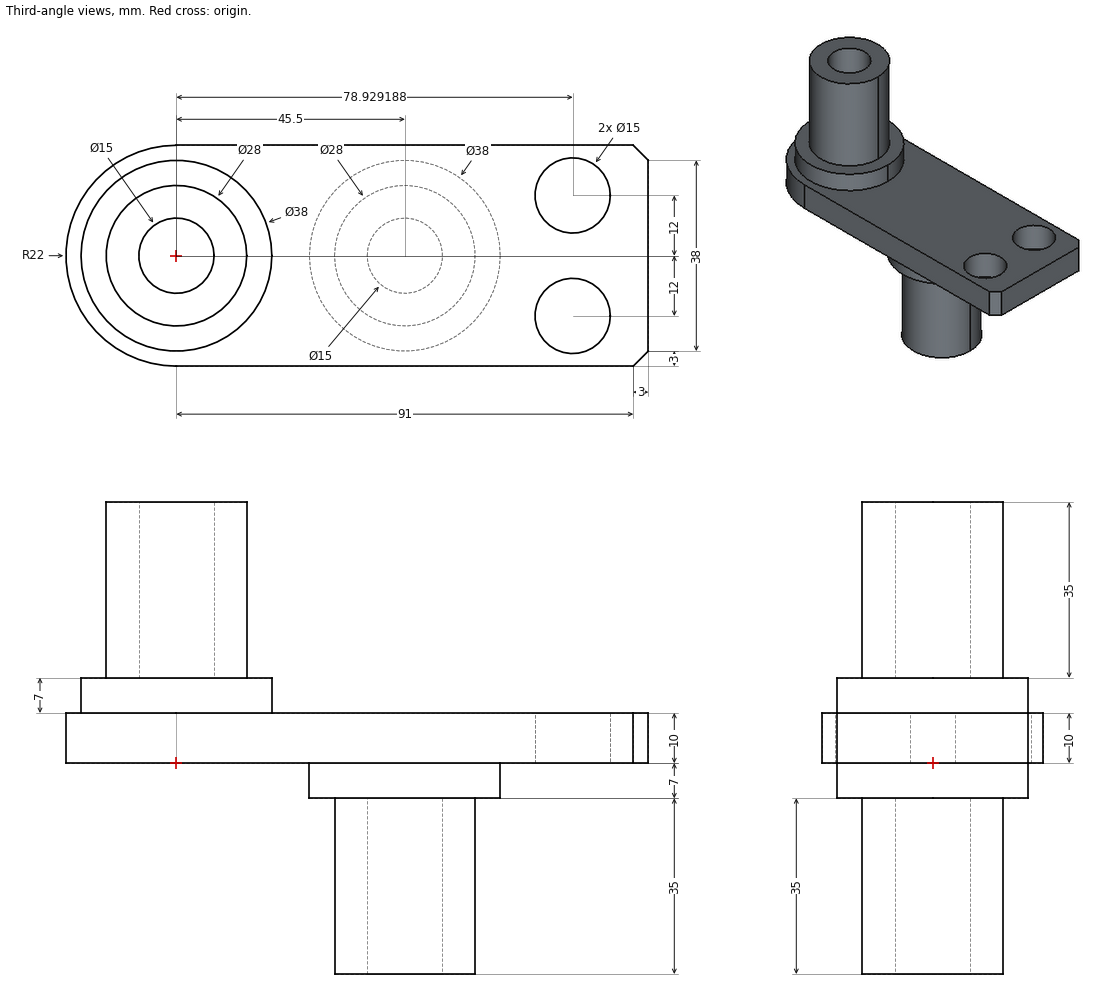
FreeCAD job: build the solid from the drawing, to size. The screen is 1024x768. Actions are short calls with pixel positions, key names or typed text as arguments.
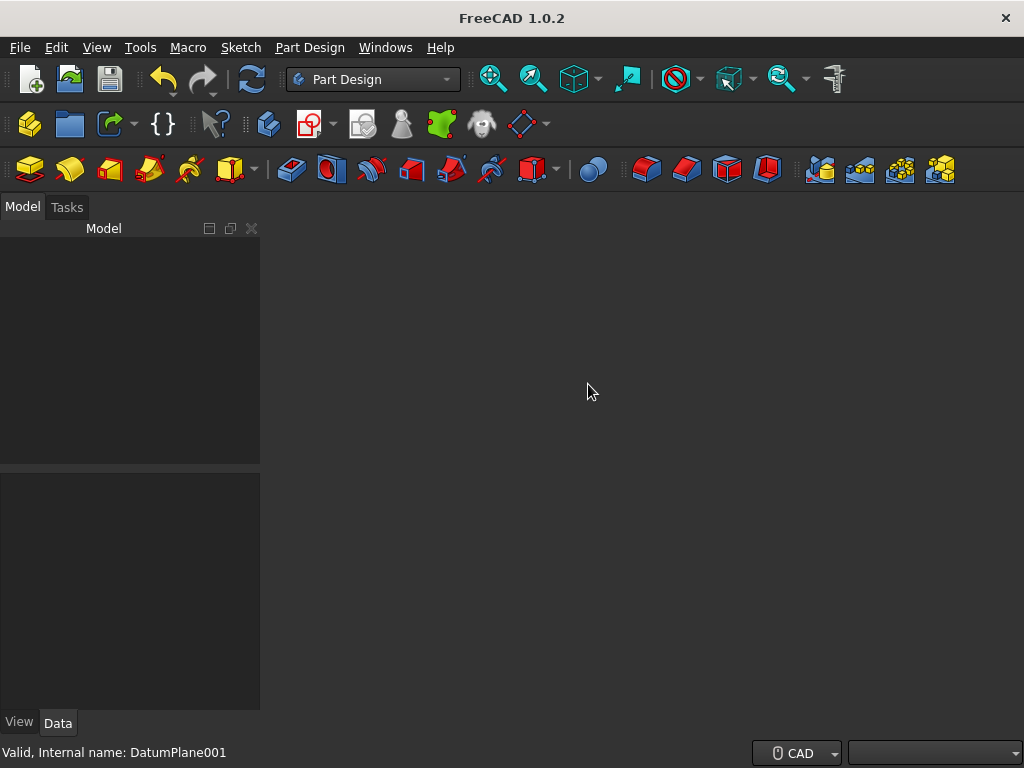
click(30, 80)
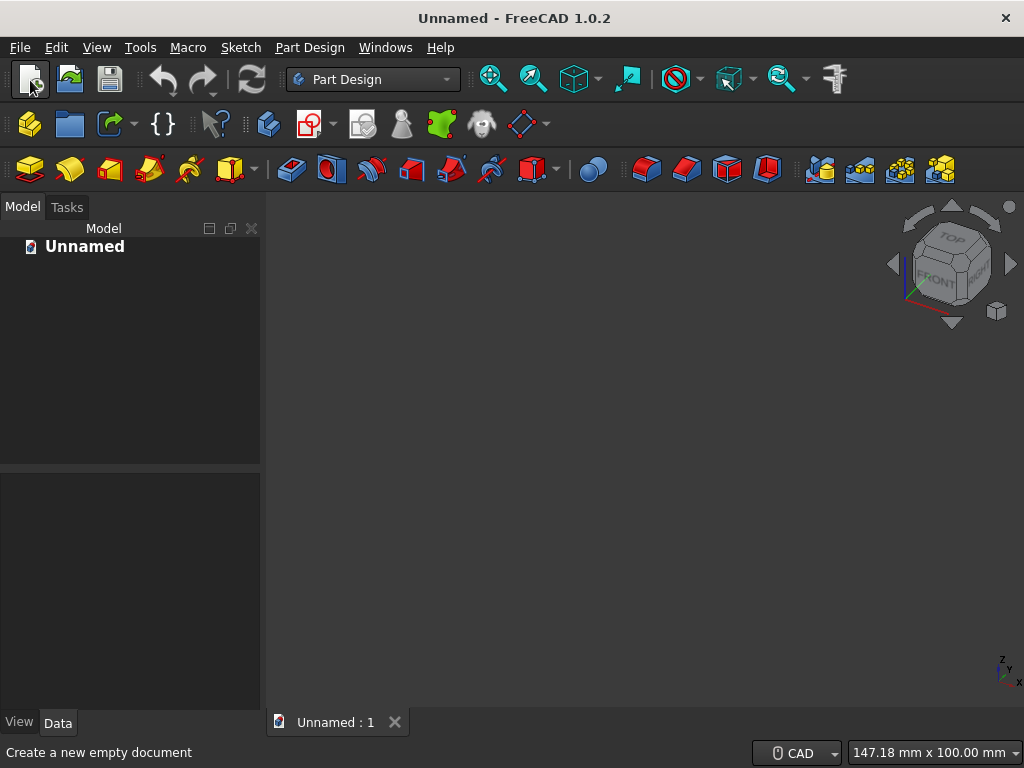
click(310, 124)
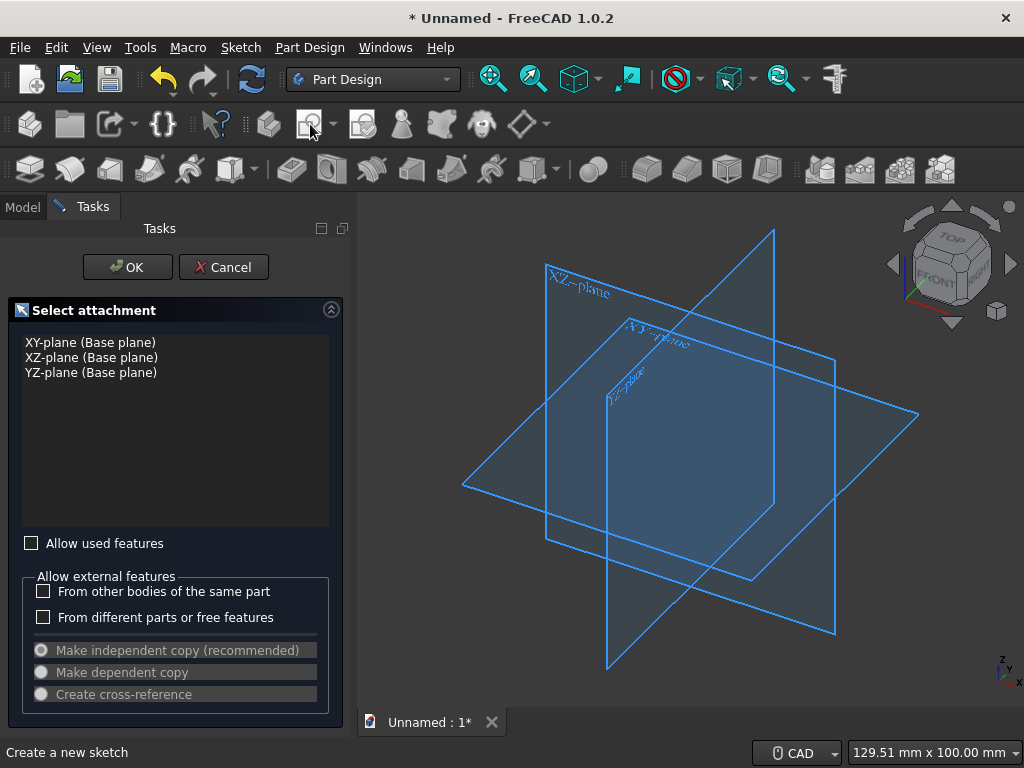
click(82, 342)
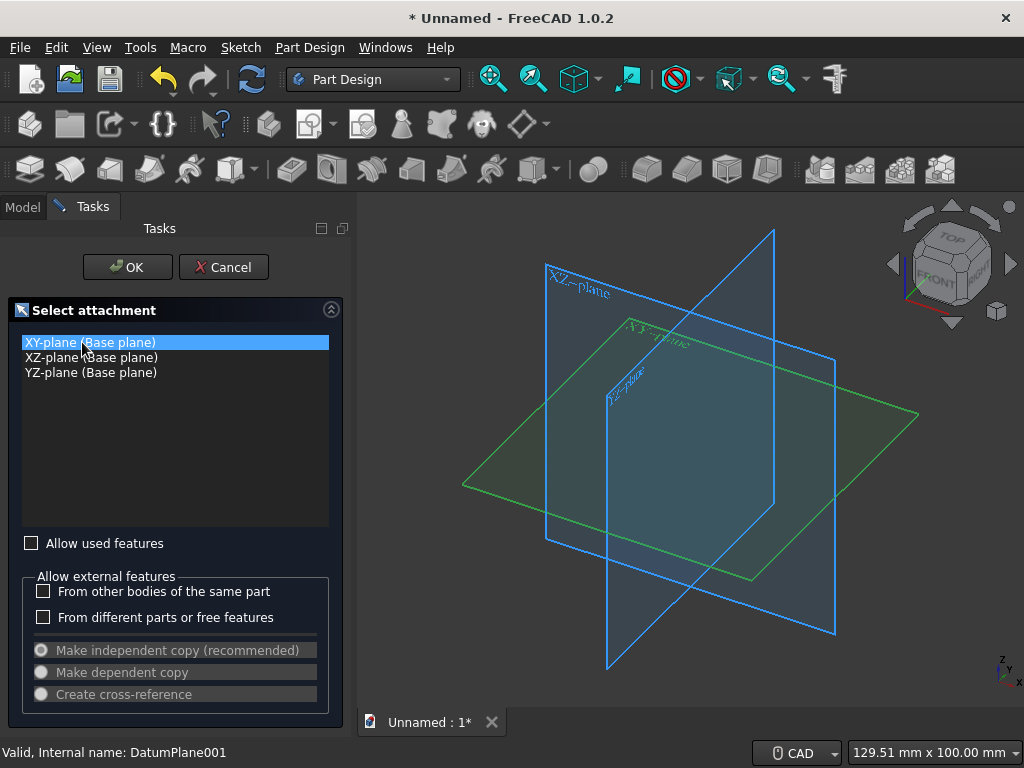
click(128, 267)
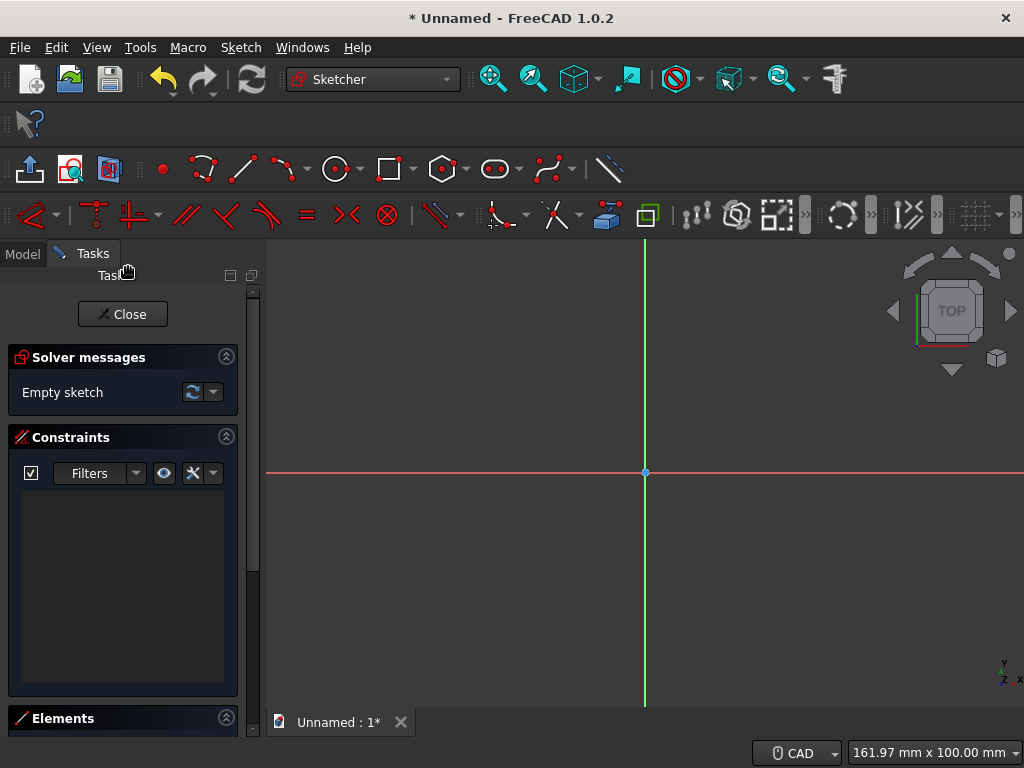
scroll(294, 473, down, 2)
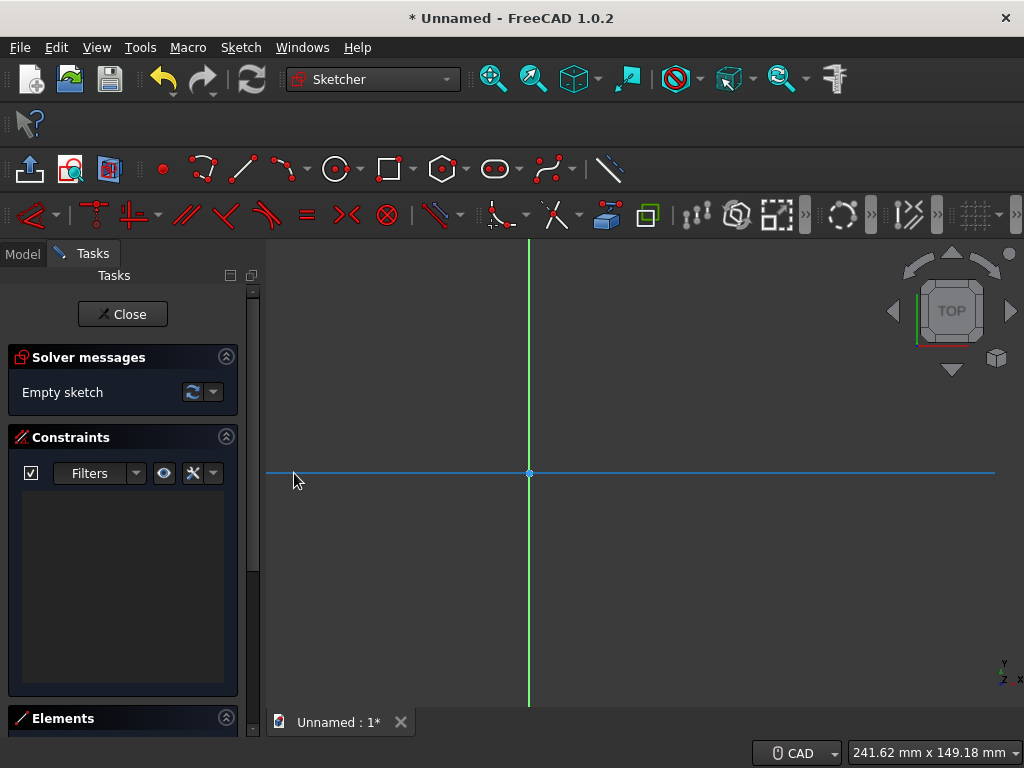
click(204, 170)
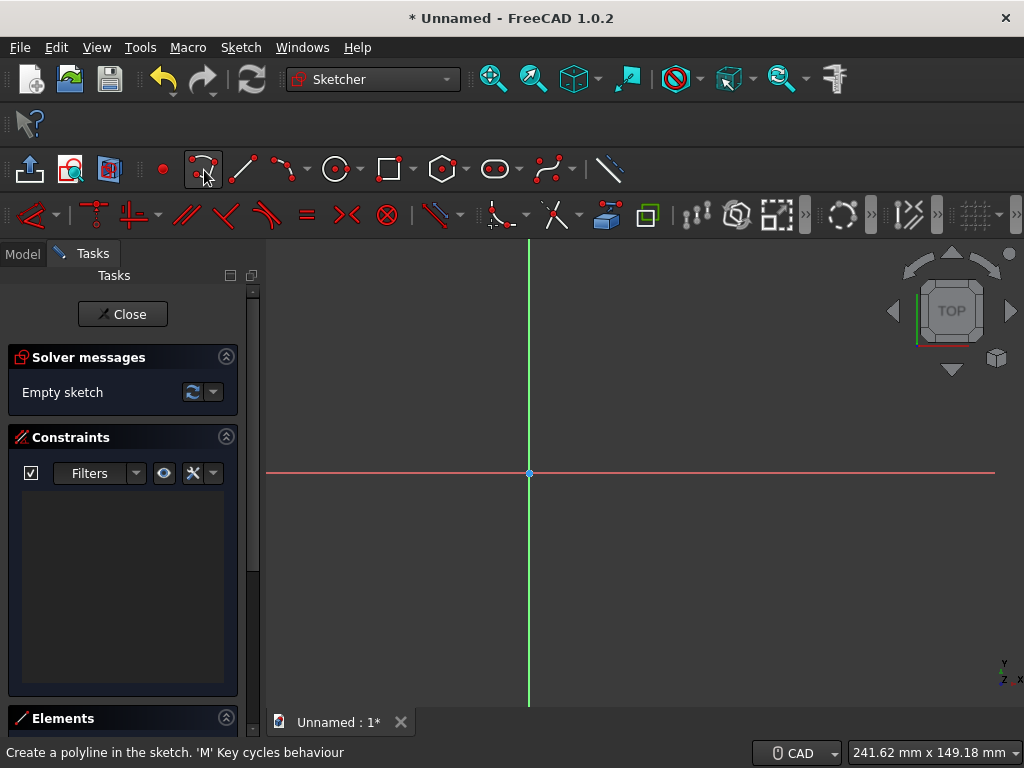
click(529, 542)
click(815, 542)
click(824, 533)
click(824, 414)
click(815, 404)
click(529, 404)
right_click(529, 404)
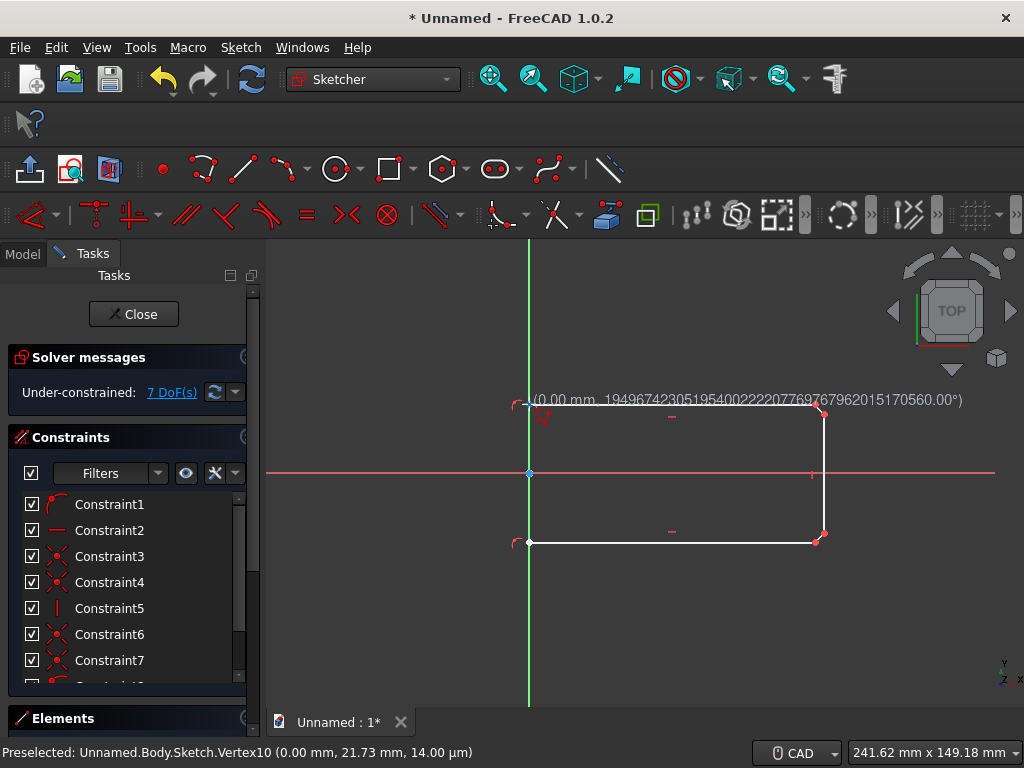
click(284, 170)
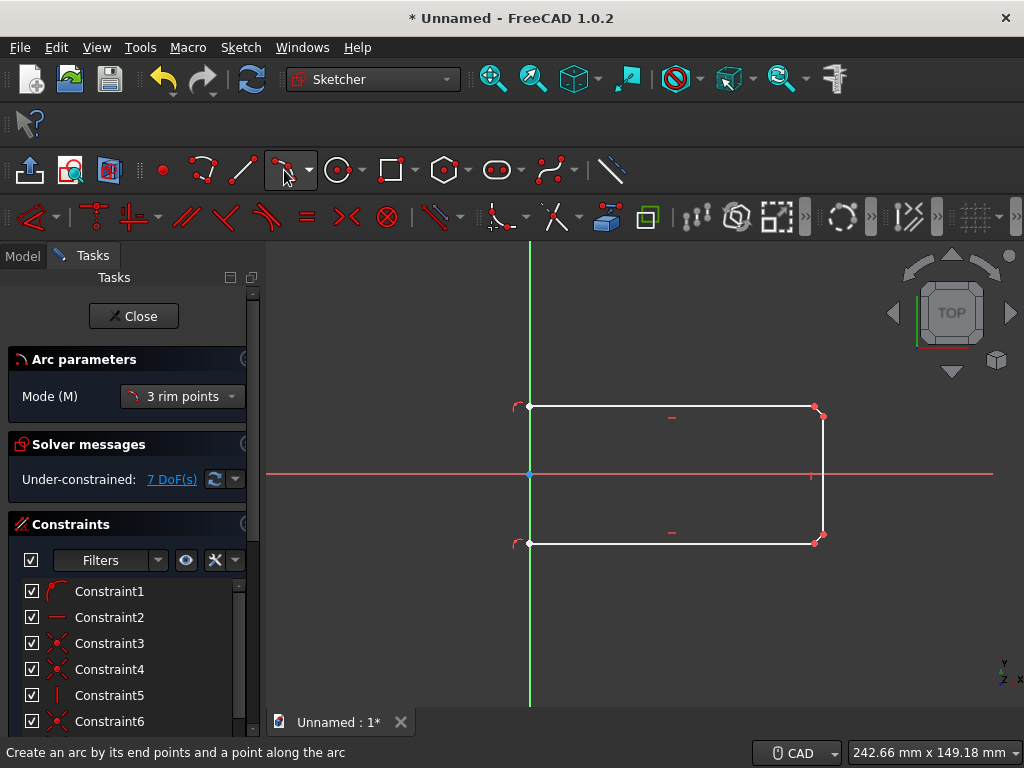
click(530, 406)
click(530, 544)
click(464, 453)
key(Escape)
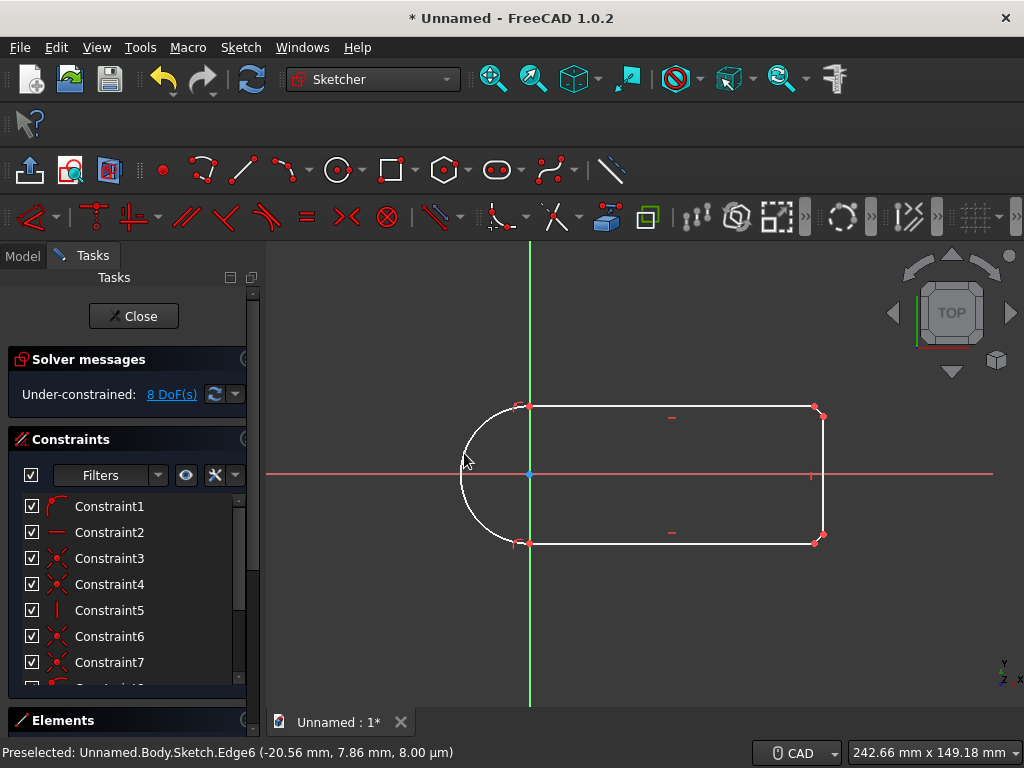
click(615, 544)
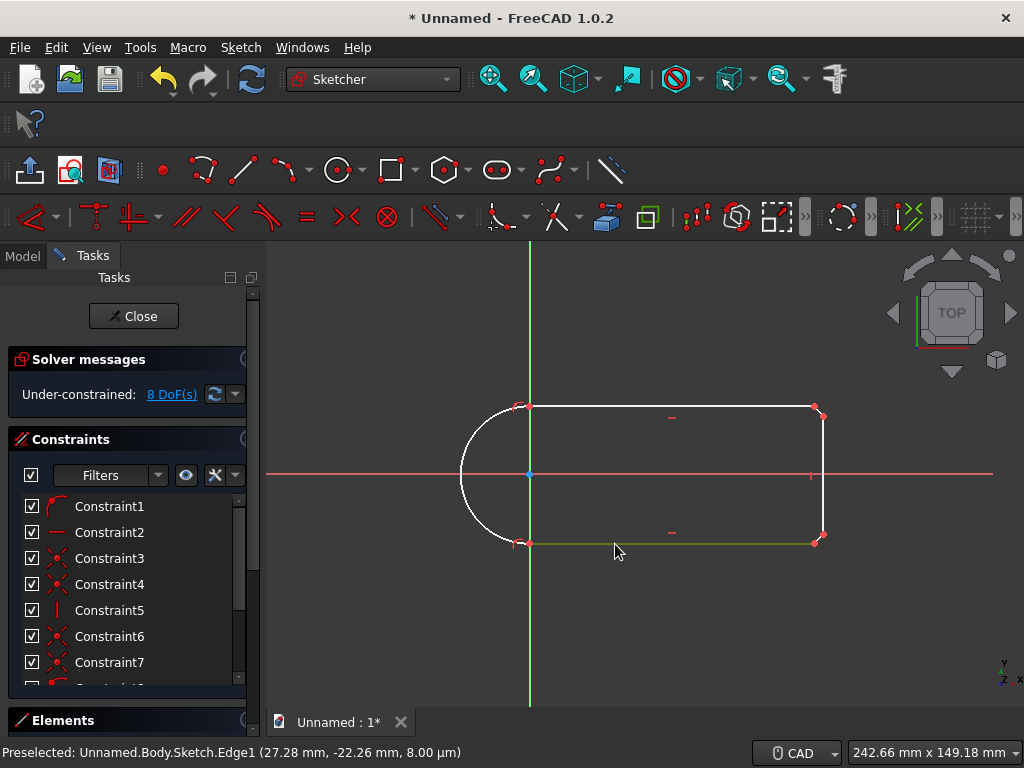
click(474, 434)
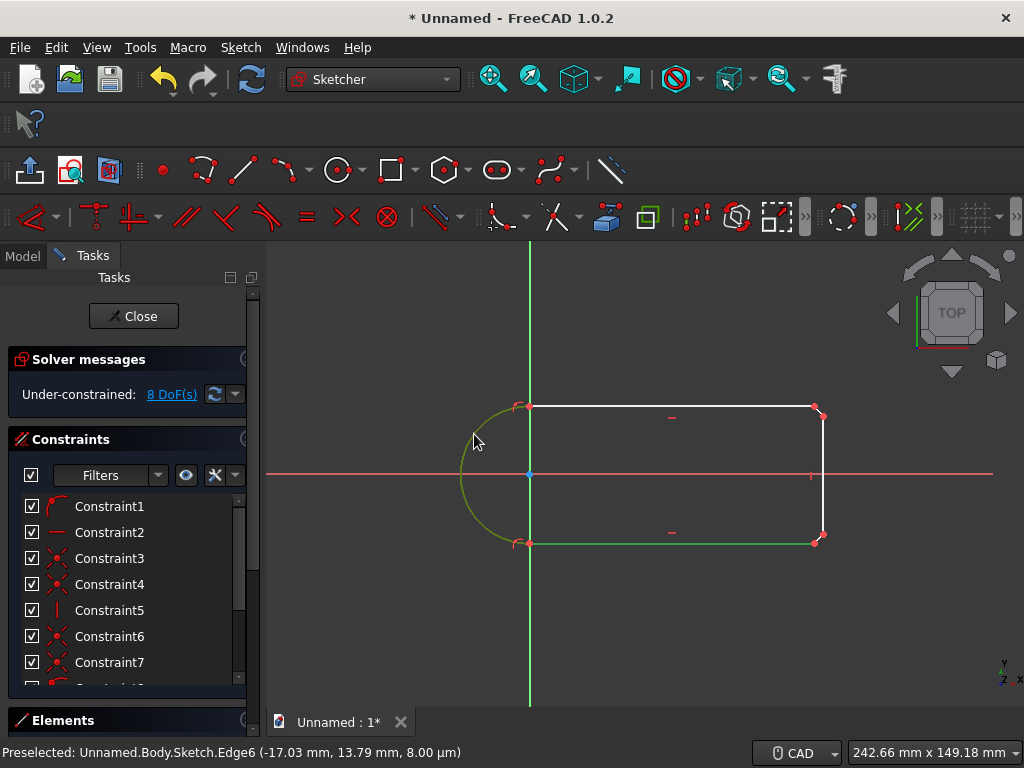
click(268, 218)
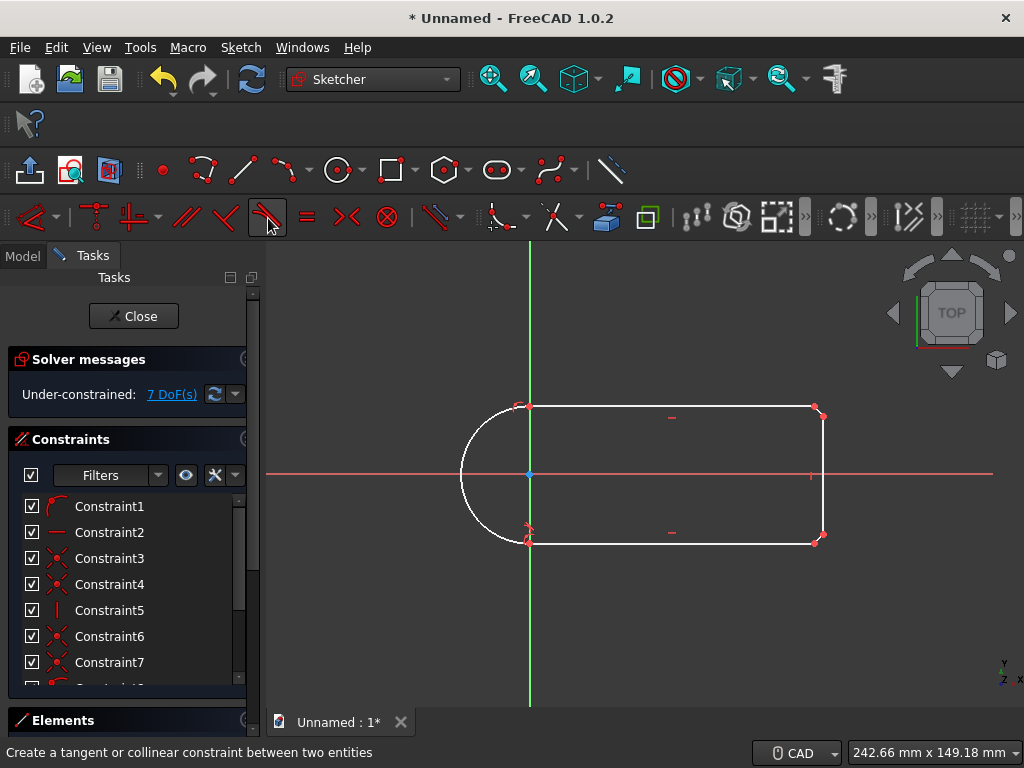
click(530, 475)